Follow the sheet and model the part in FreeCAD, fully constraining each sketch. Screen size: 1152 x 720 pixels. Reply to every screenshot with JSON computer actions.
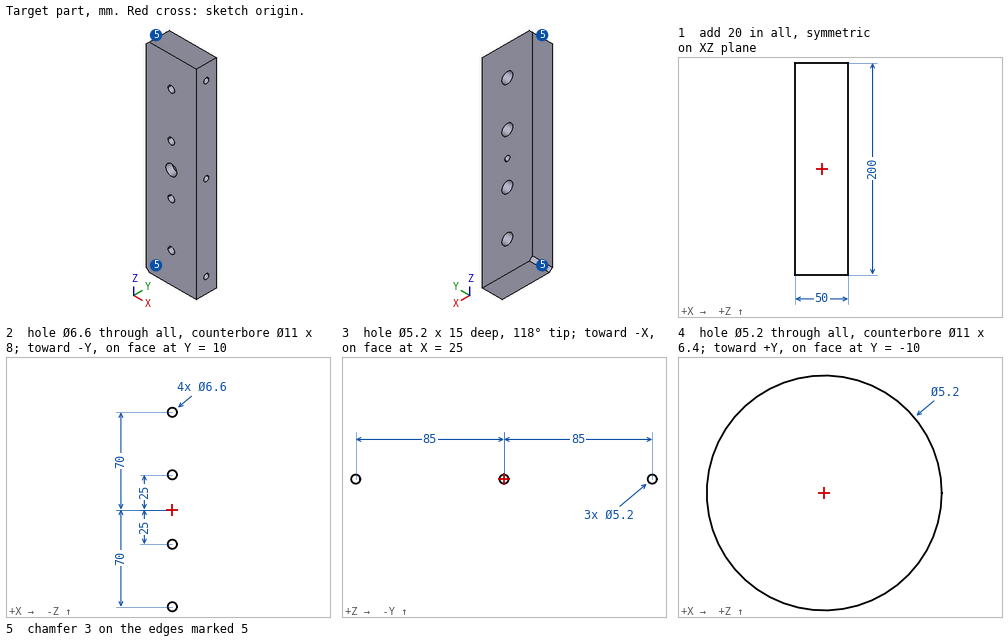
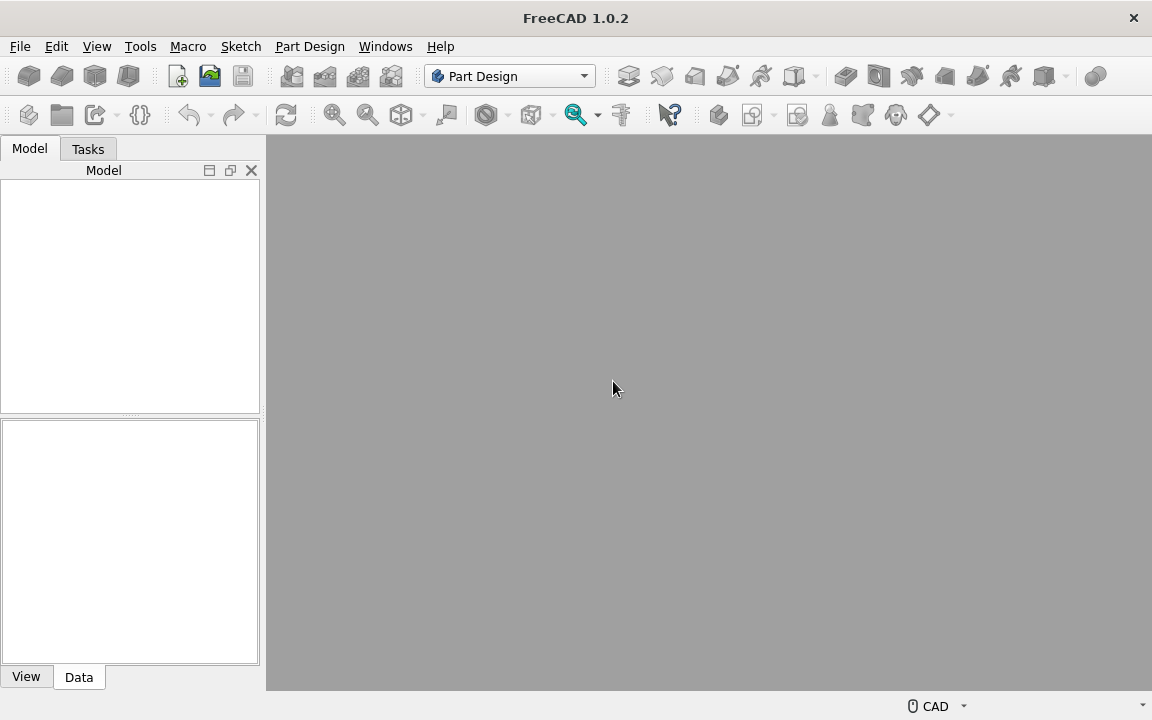
{"action": "left_click", "coordinate": [177, 76]}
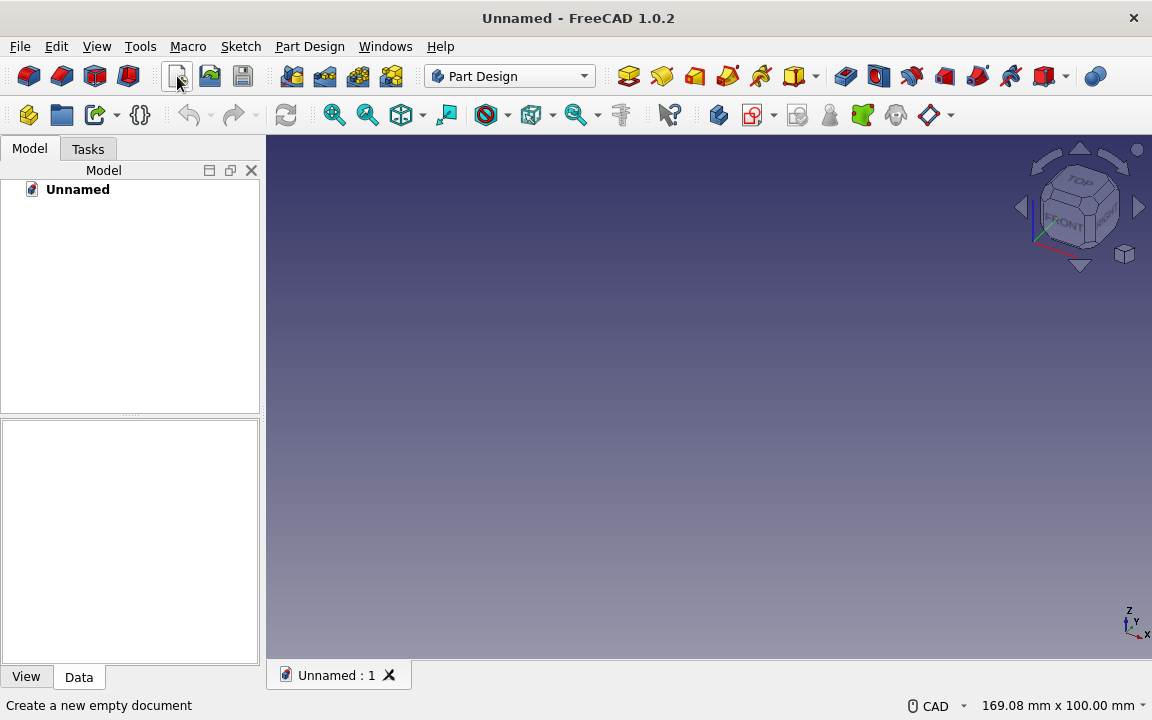
{"action": "left_click", "coordinate": [752, 116]}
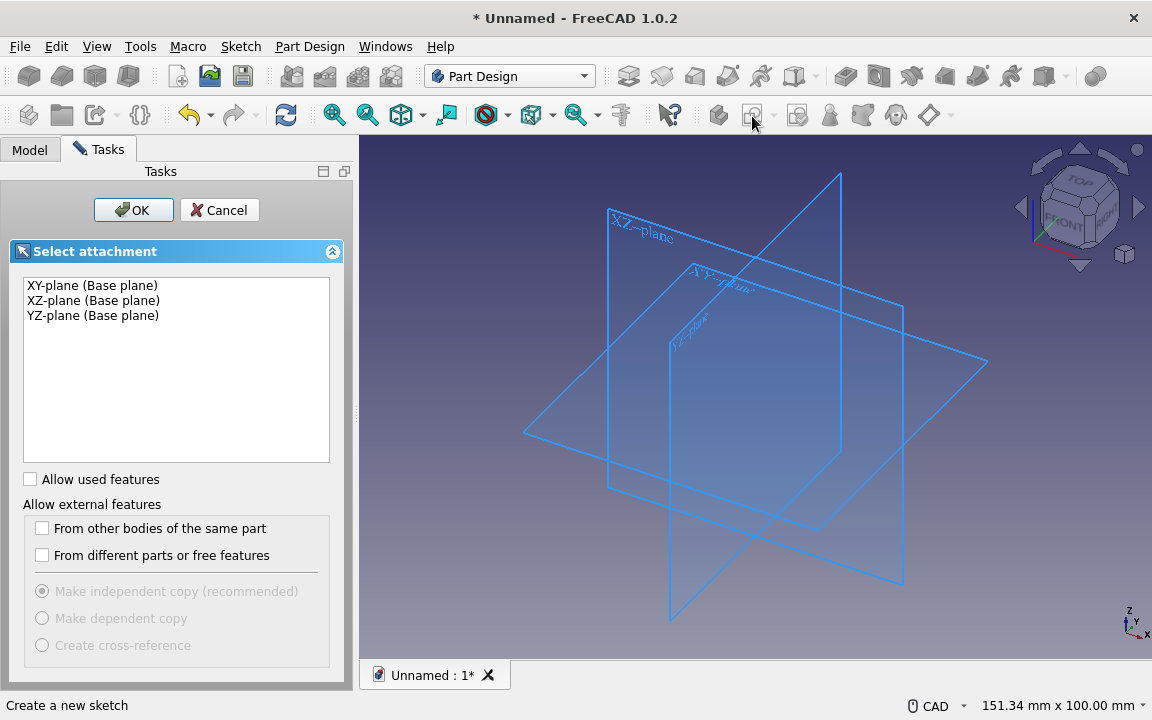
{"action": "left_click", "coordinate": [84, 300]}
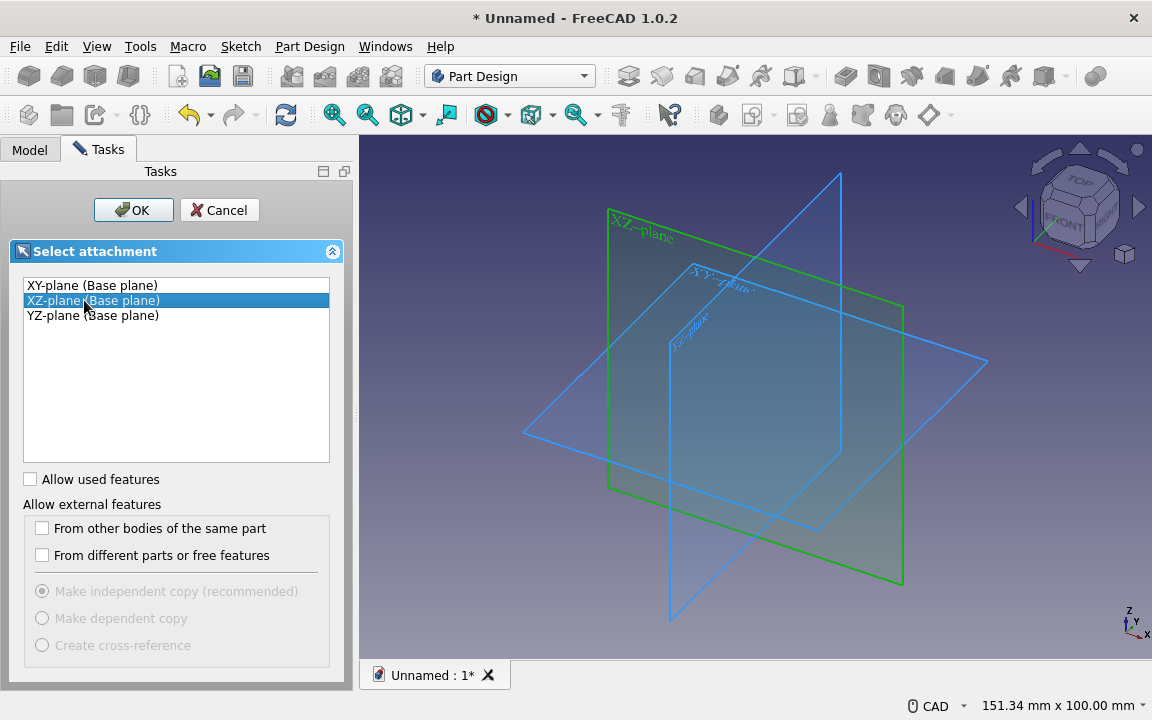
{"action": "left_click", "coordinate": [134, 210]}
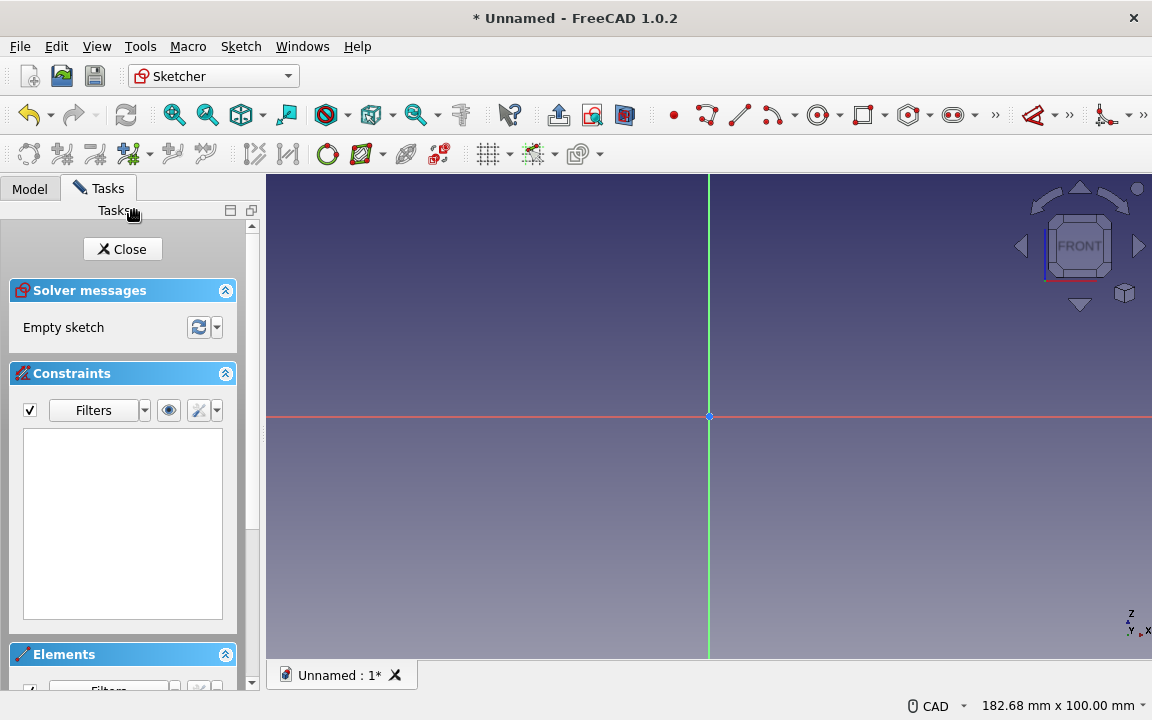
{"action": "scroll", "coordinate": [611, 416], "scroll_direction": "down", "scroll_amount": 6}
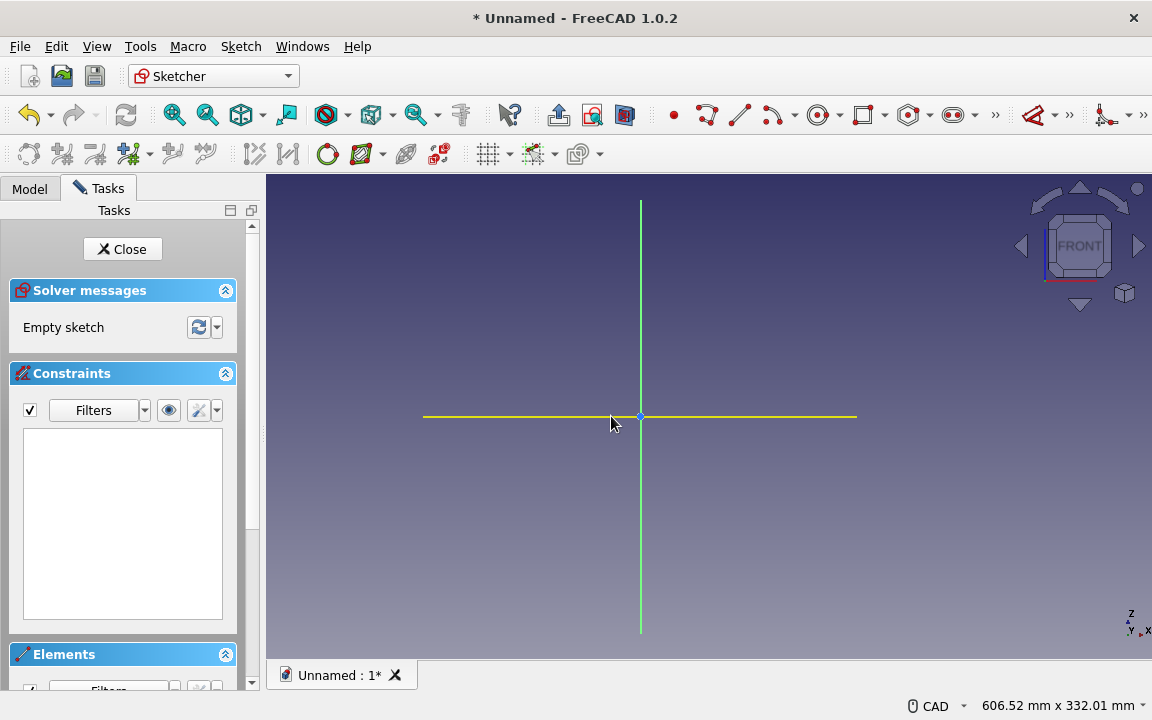
{"action": "left_click", "coordinate": [884, 116]}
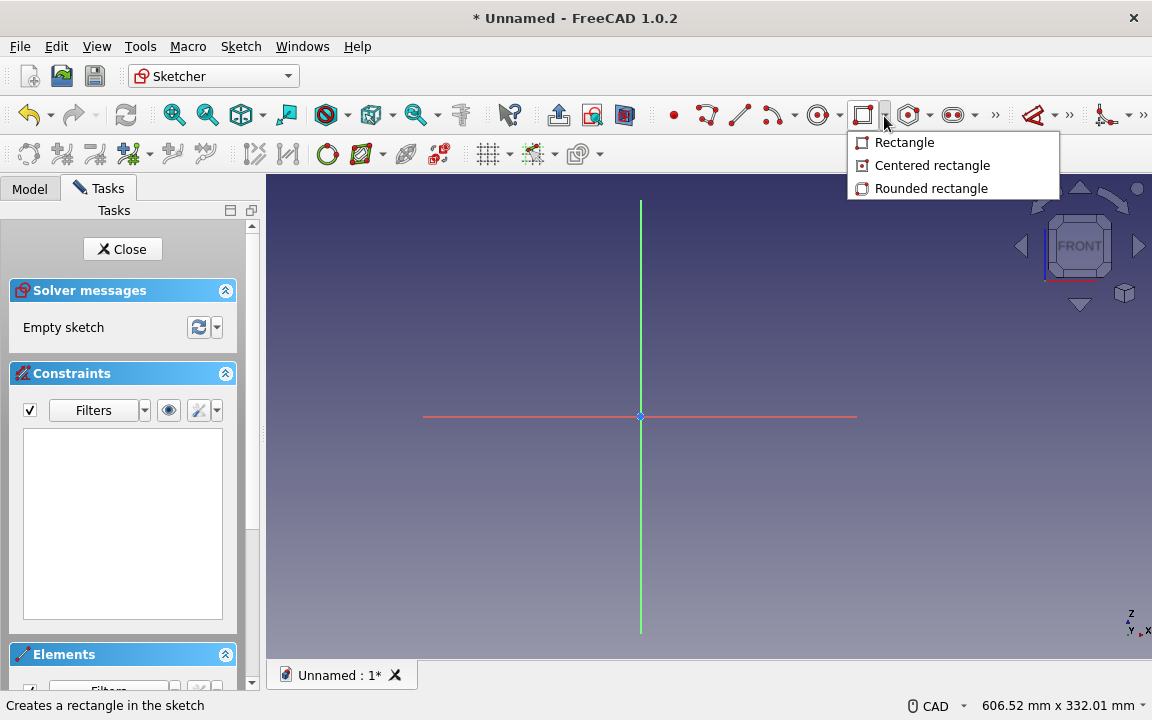
{"action": "left_click", "coordinate": [954, 166]}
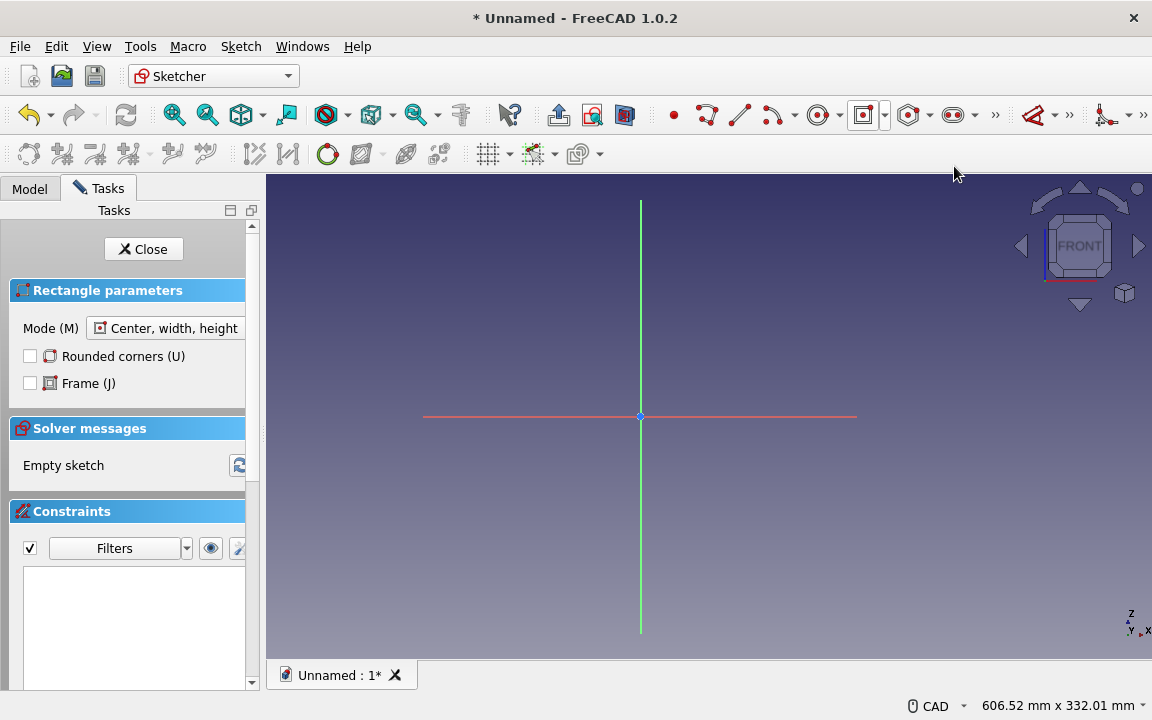
{"action": "left_click", "coordinate": [641, 416]}
{"action": "left_click", "coordinate": [677, 270]}
{"action": "key", "text": "Escape"}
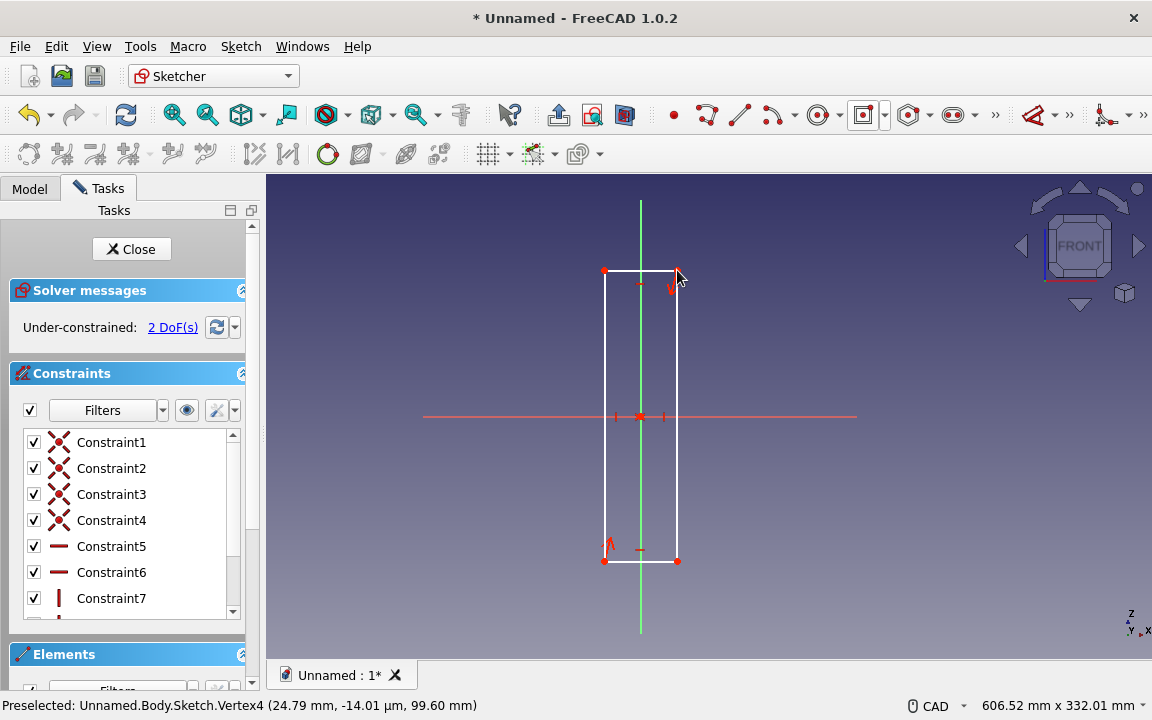
{"action": "left_click", "coordinate": [626, 562]}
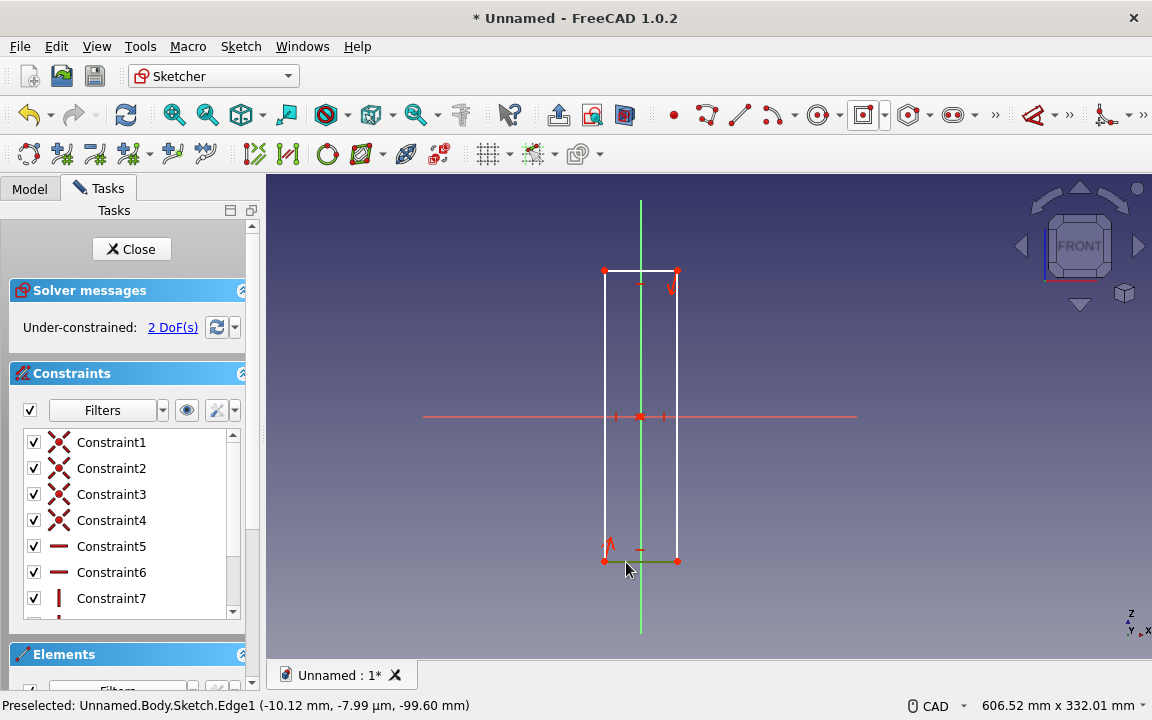
{"action": "left_click", "coordinate": [1054, 116]}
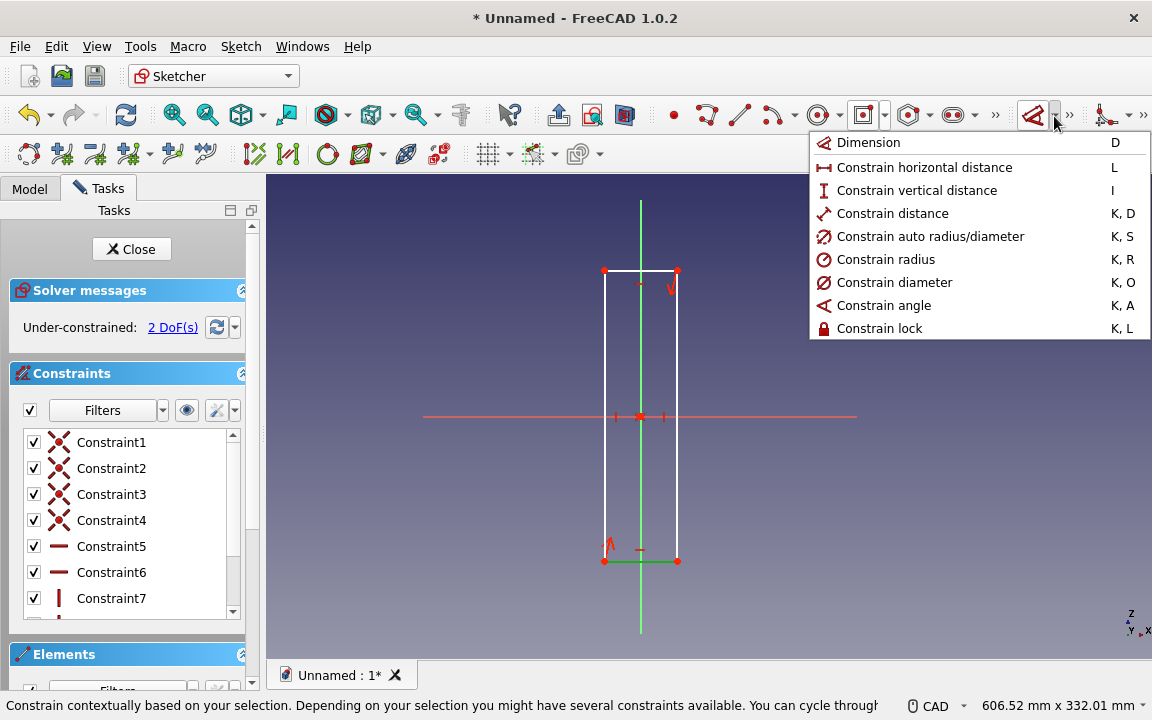
{"action": "left_click", "coordinate": [980, 168]}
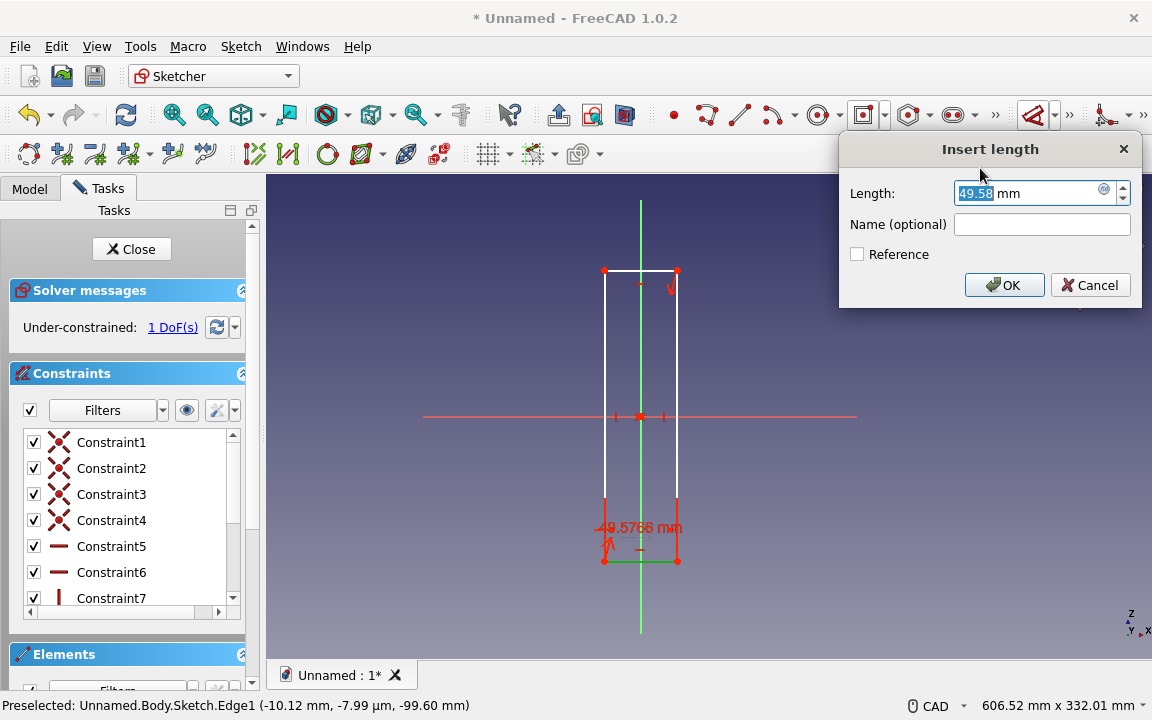
{"action": "type", "text": "50"}
{"action": "key", "text": "Return"}